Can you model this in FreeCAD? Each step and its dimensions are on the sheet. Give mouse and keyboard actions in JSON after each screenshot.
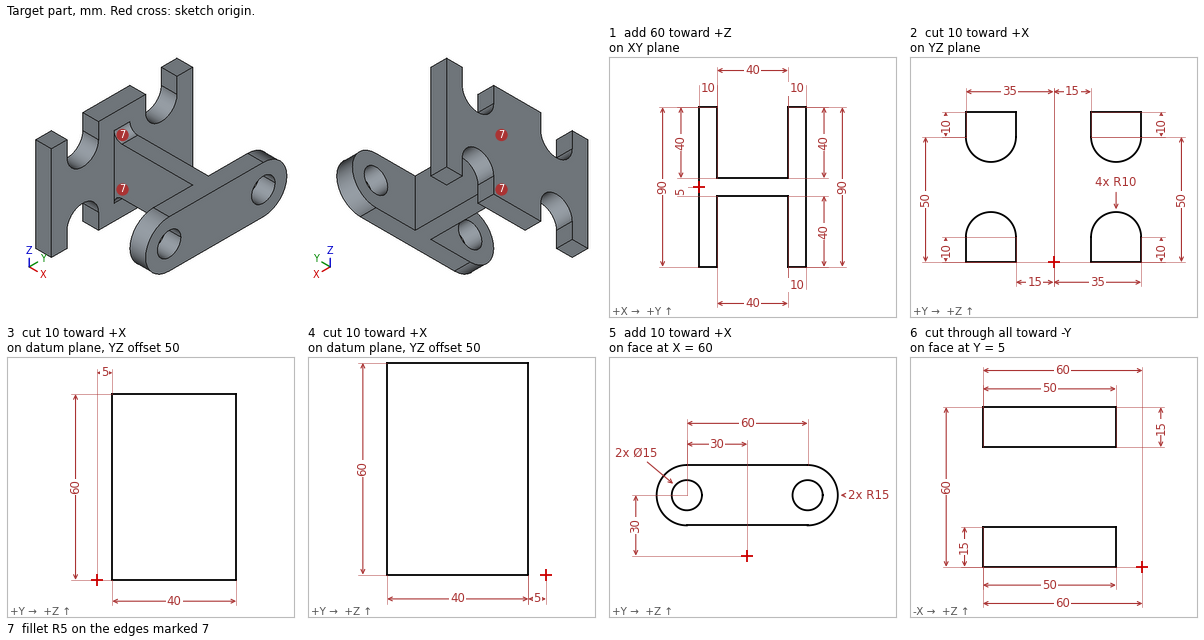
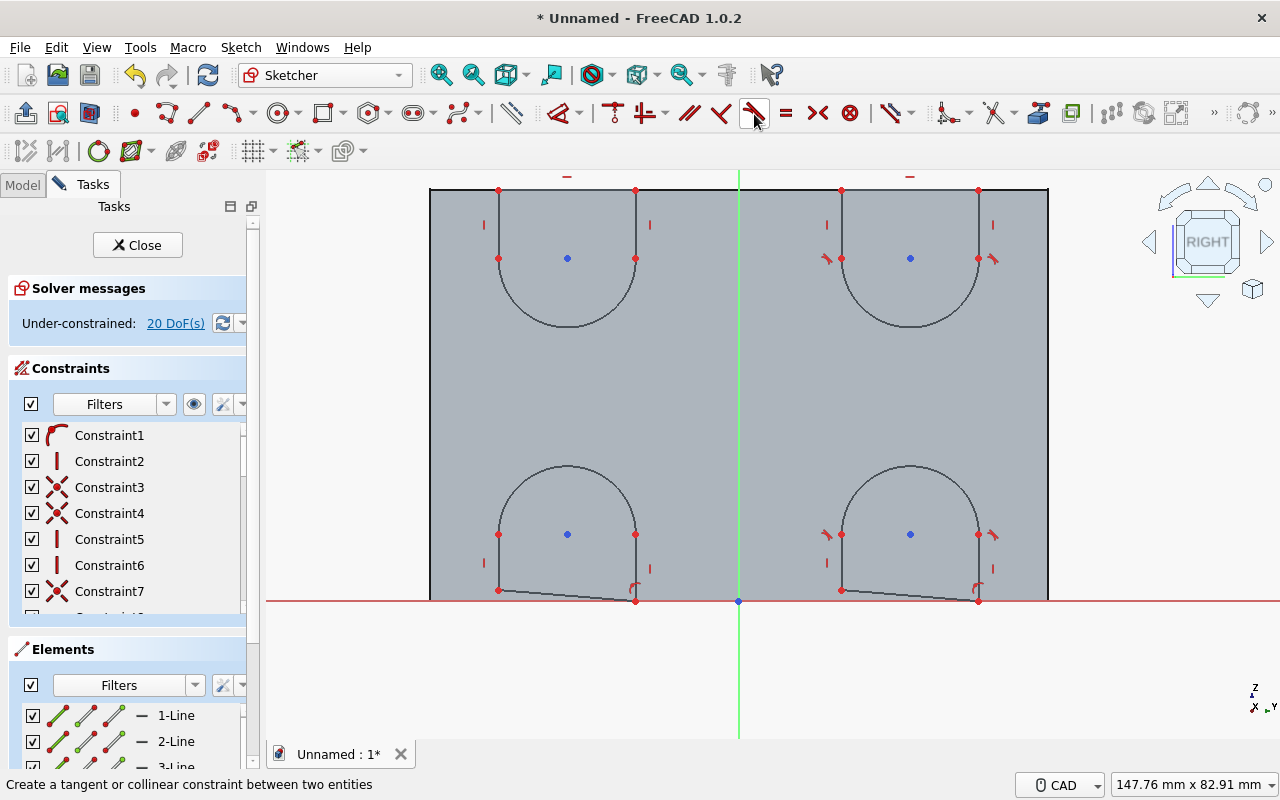
{"action": "left_click", "coordinate": [636, 555]}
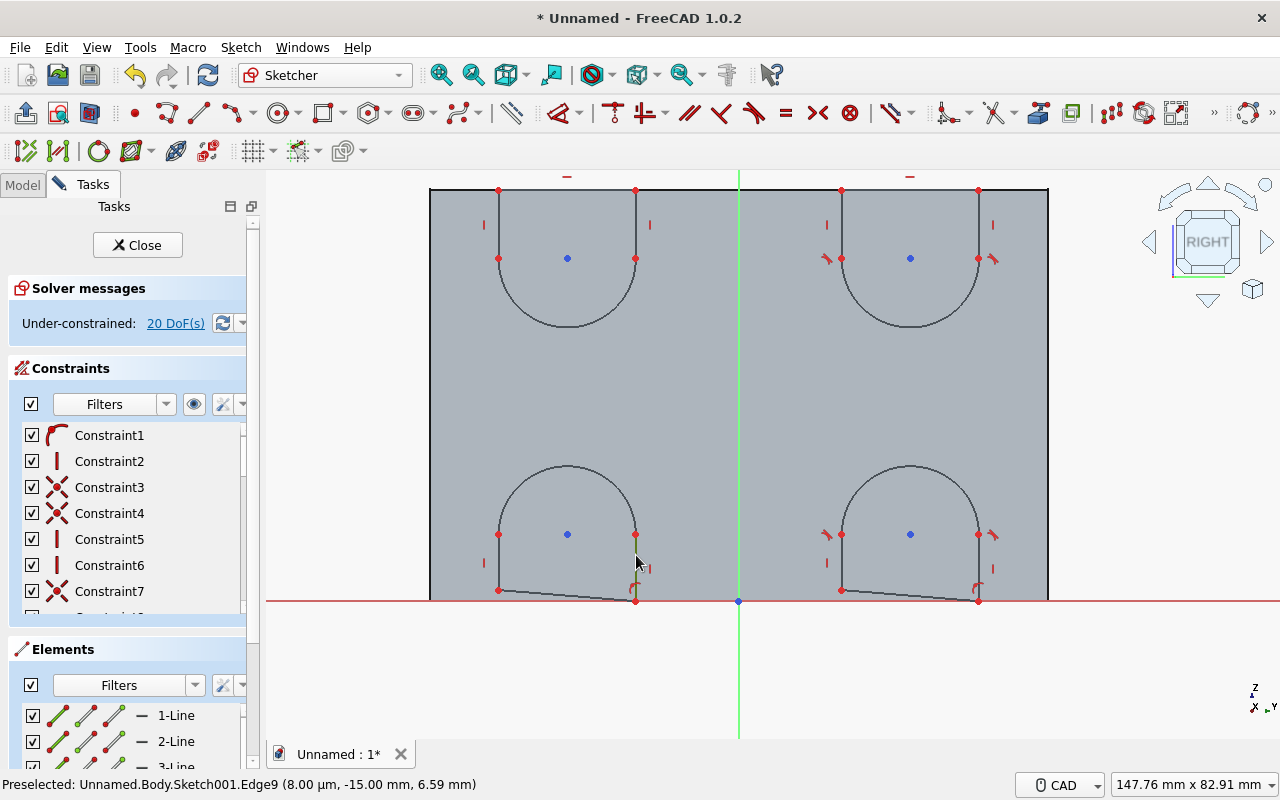
{"action": "left_click", "coordinate": [608, 479]}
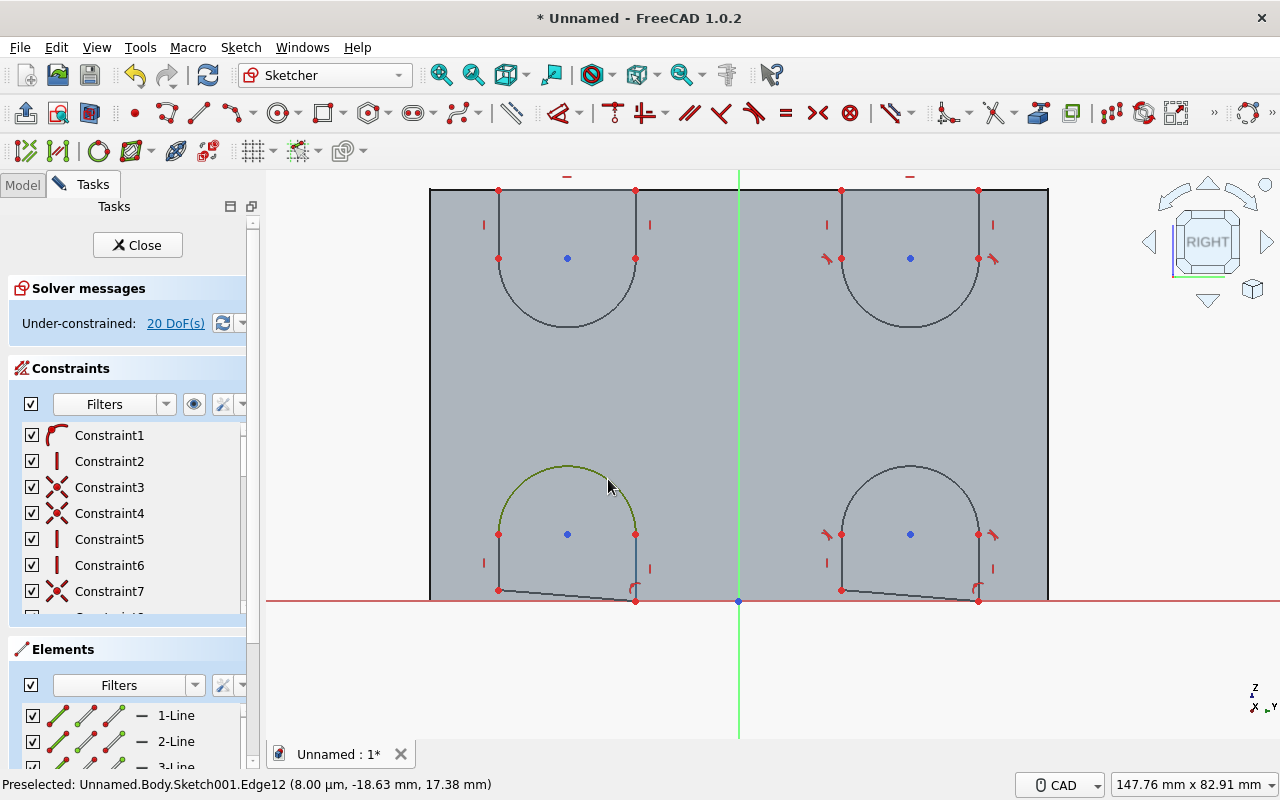
{"action": "left_click", "coordinate": [754, 114]}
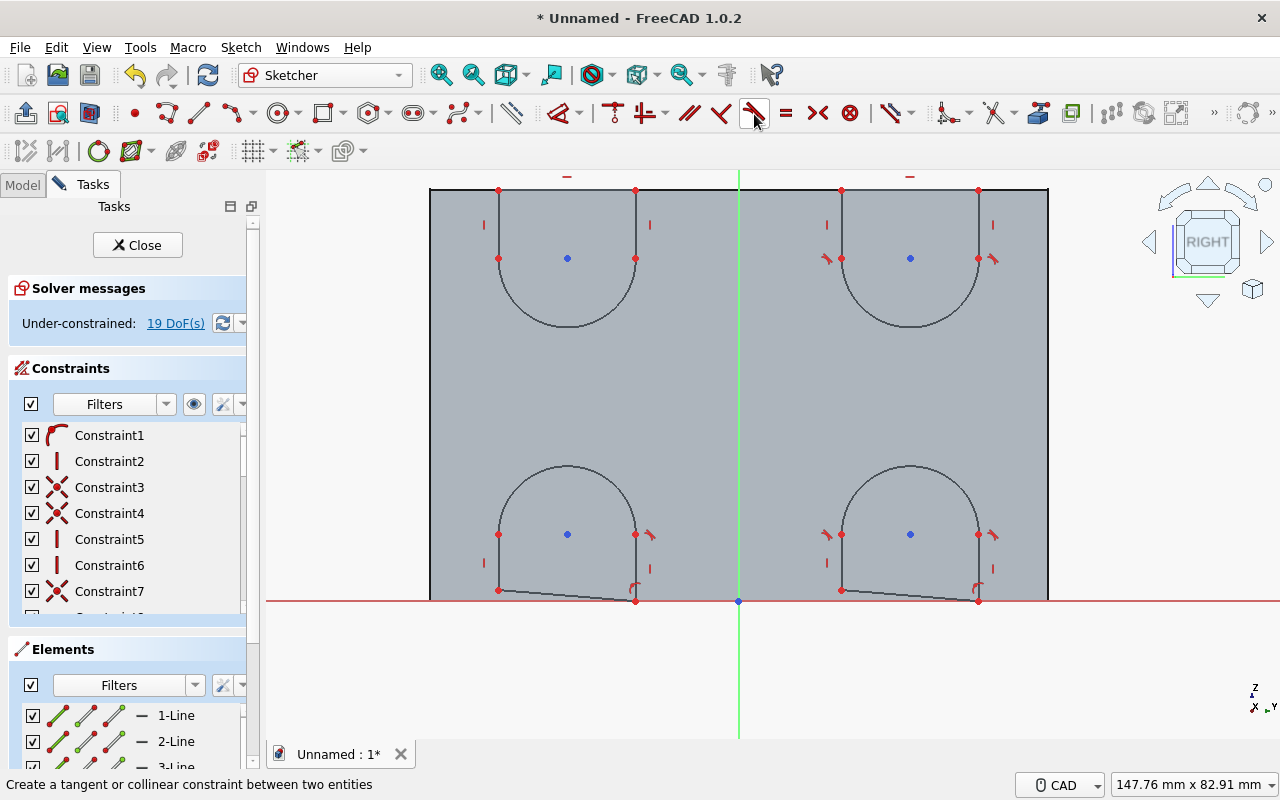
{"action": "left_click", "coordinate": [499, 574]}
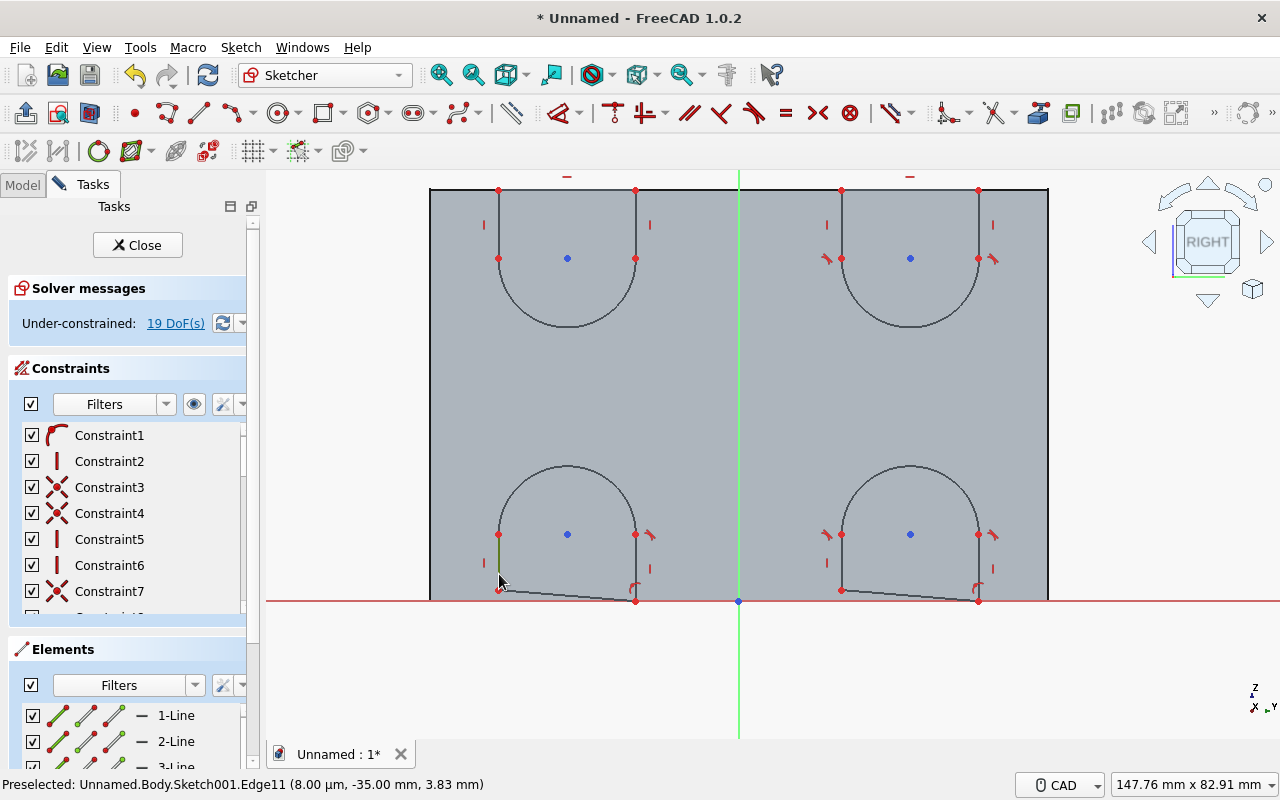
{"action": "left_click", "coordinate": [608, 479]}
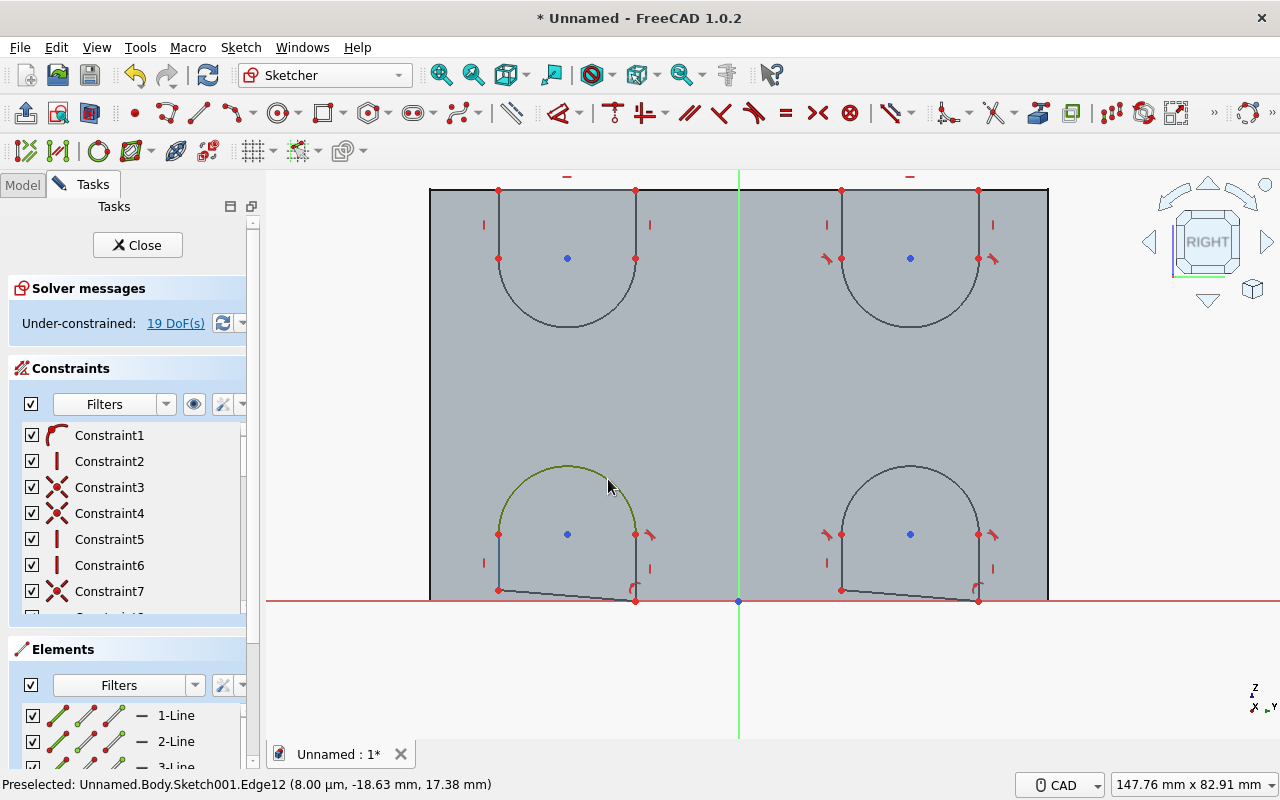
{"action": "left_click", "coordinate": [754, 114]}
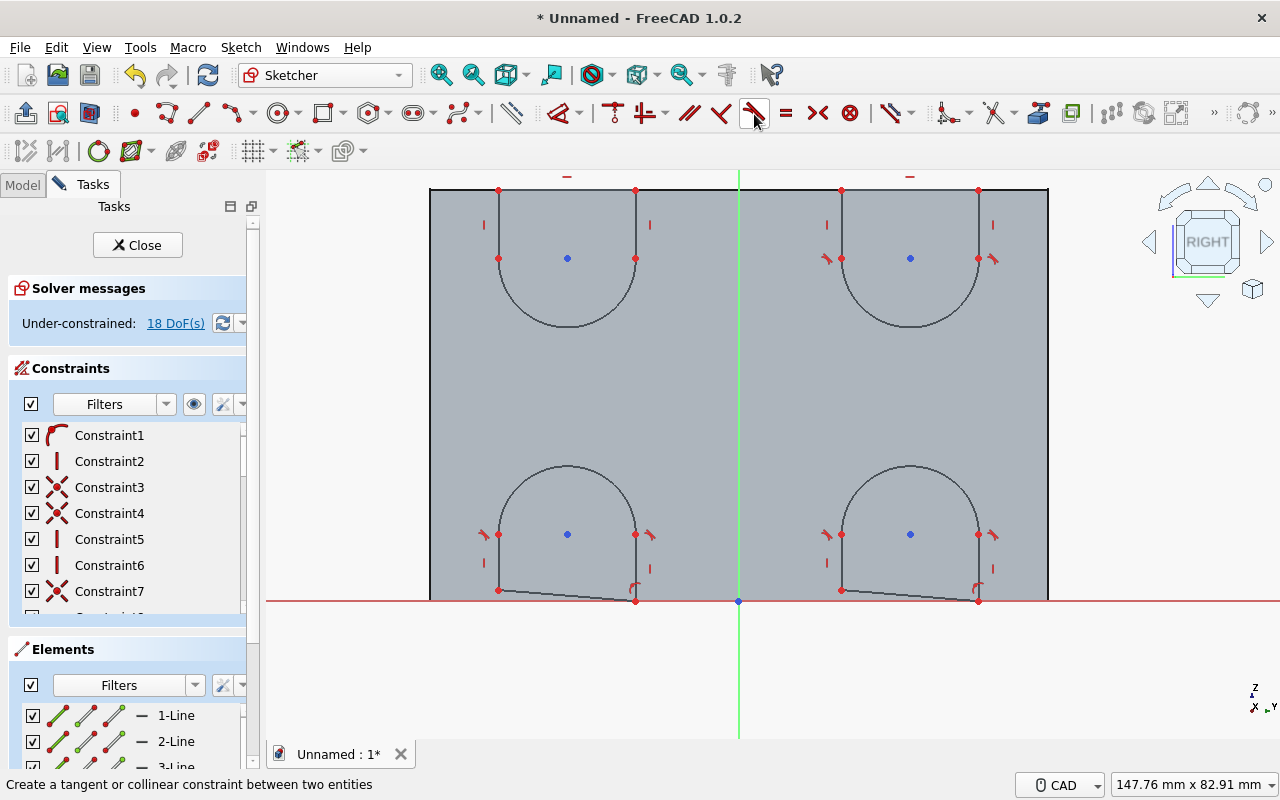
{"action": "left_click", "coordinate": [499, 238]}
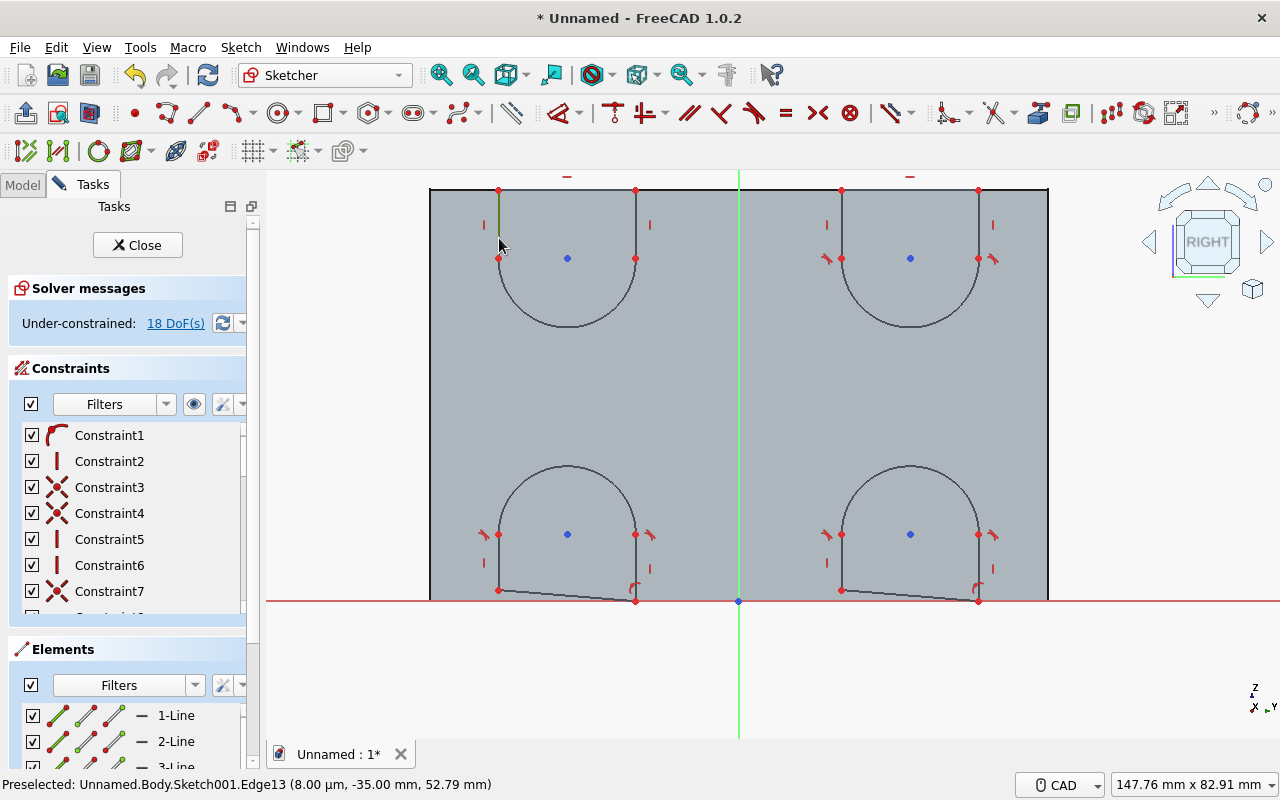
{"action": "left_click", "coordinate": [527, 314]}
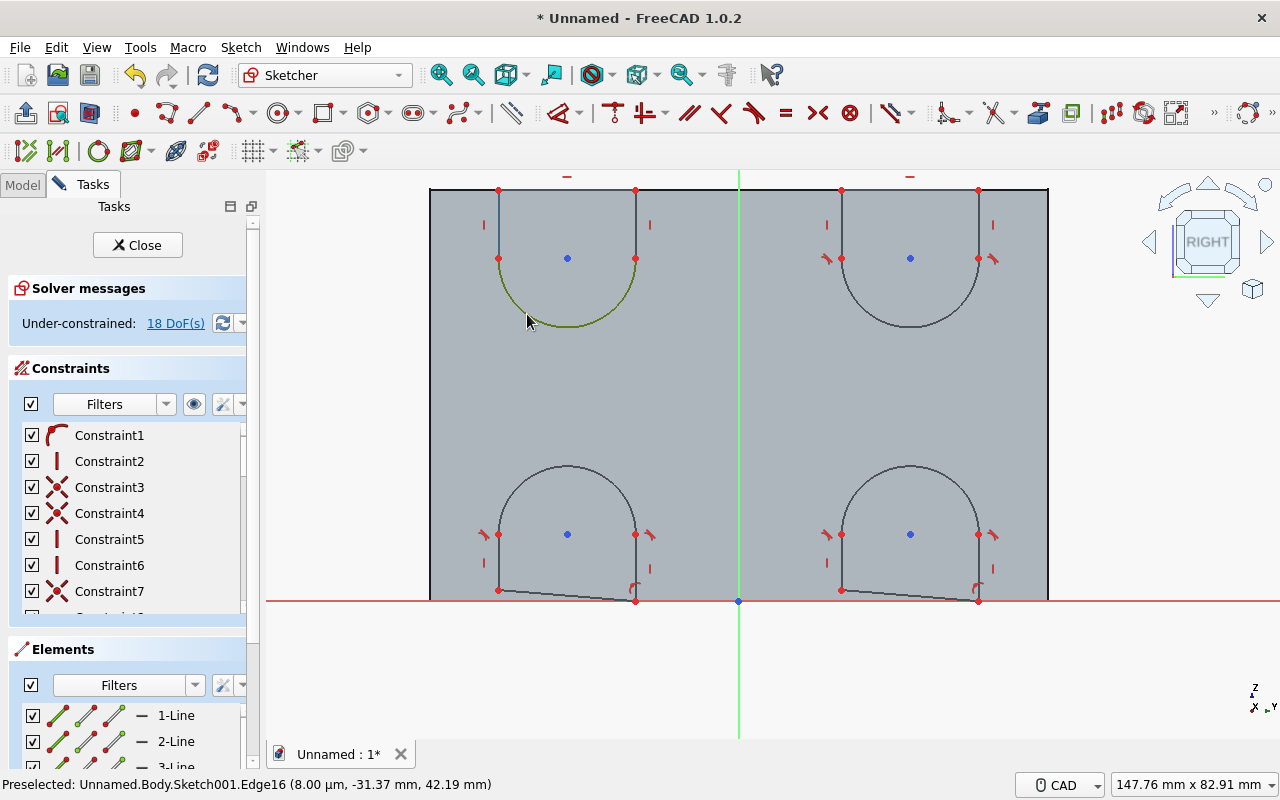
{"action": "left_click", "coordinate": [754, 114]}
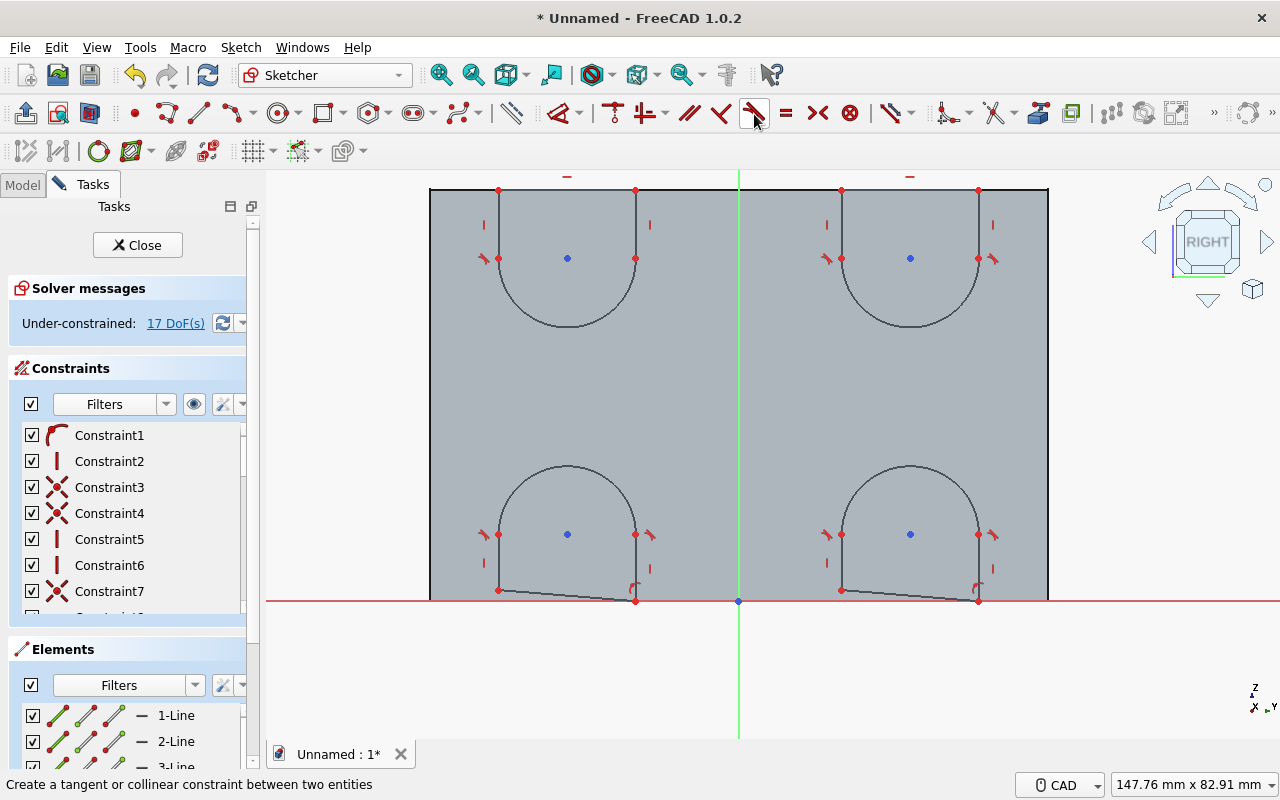
{"action": "left_click", "coordinate": [636, 211]}